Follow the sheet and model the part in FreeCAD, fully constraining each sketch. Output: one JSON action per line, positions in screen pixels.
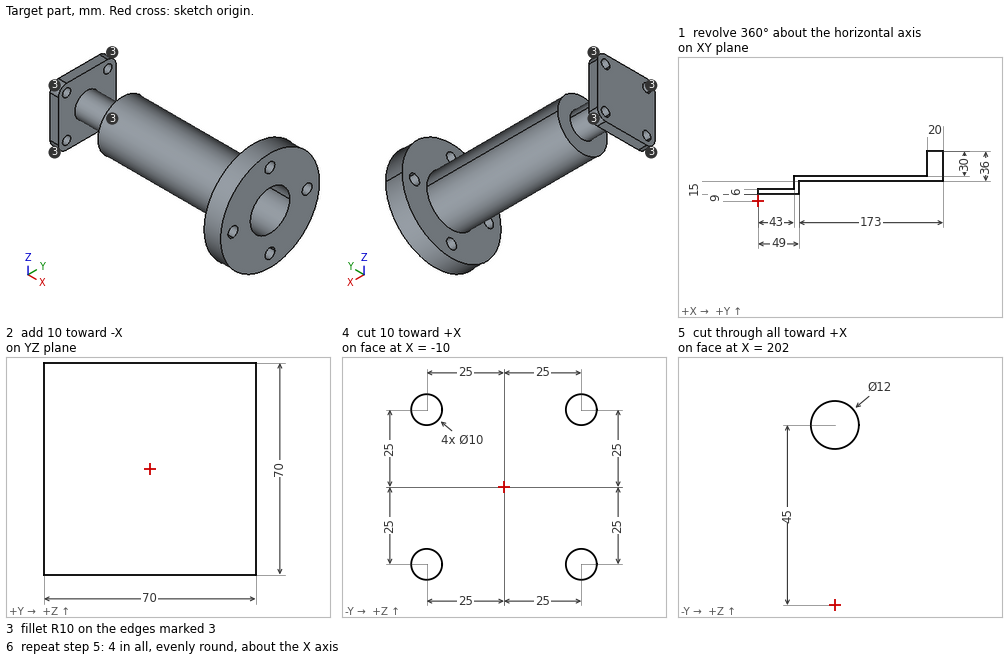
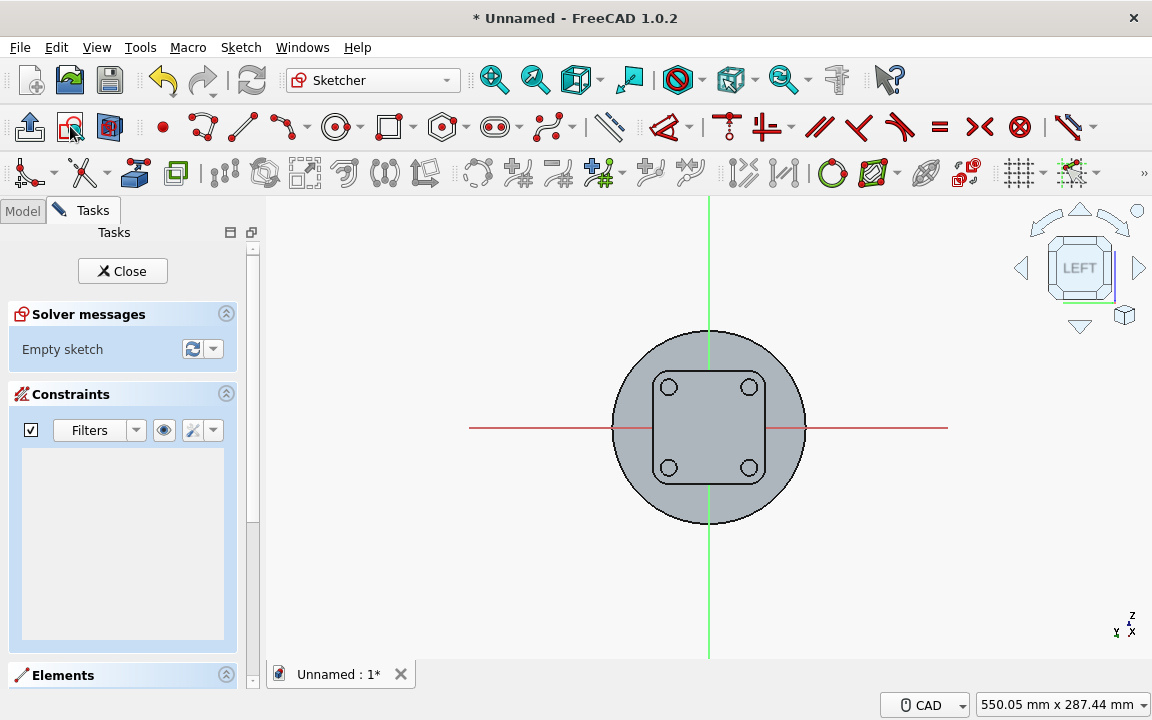
{"action": "scroll", "coordinate": [714, 349], "scroll_direction": "up", "scroll_amount": 13}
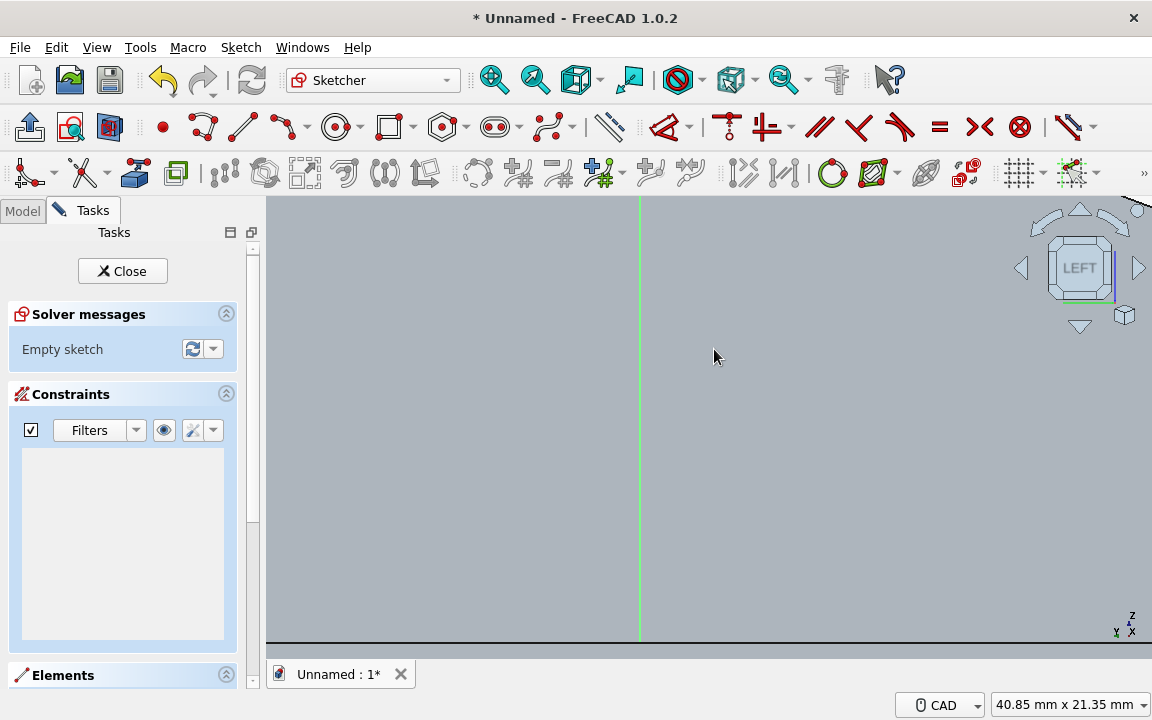
{"action": "key", "text": "g c"}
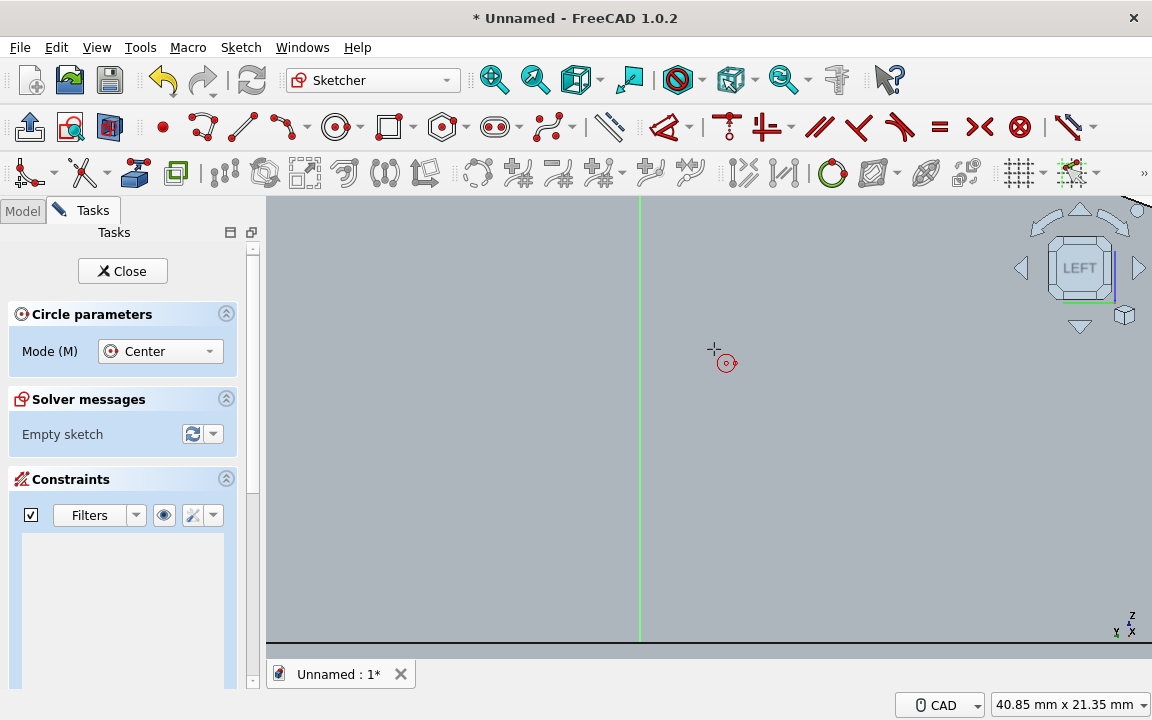
{"action": "left_click", "coordinate": [640, 426]}
{"action": "mouse_move", "coordinate": [732, 334]}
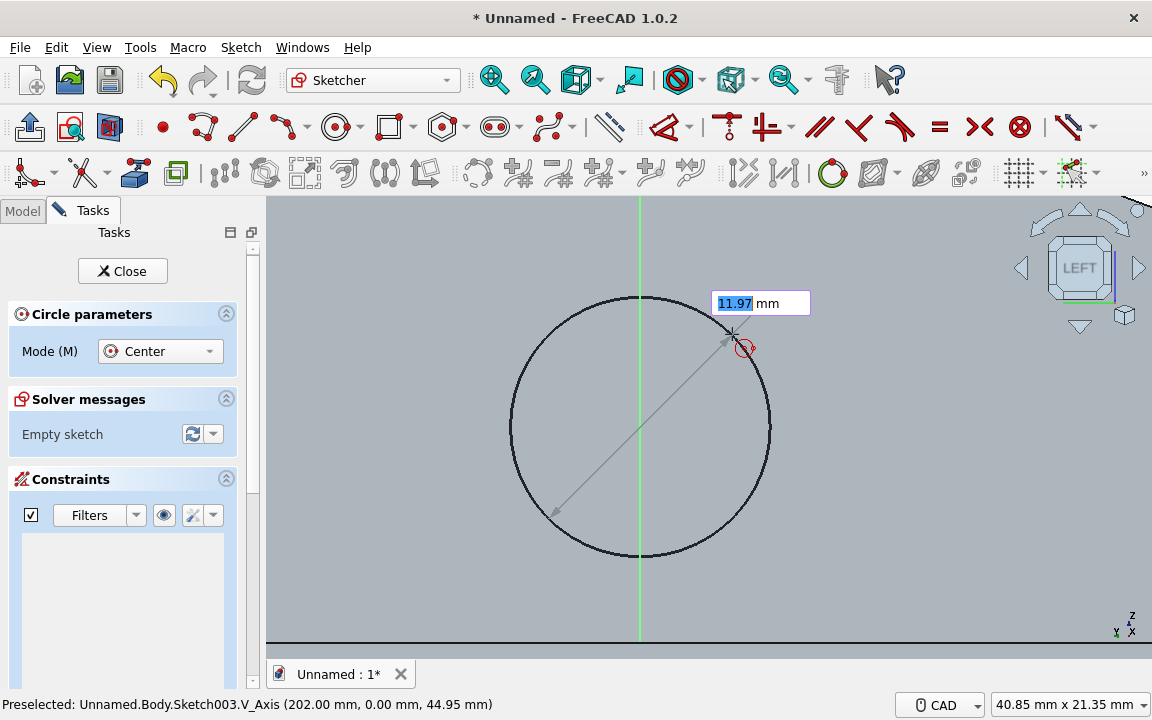
{"action": "type", "text": "12"}
{"action": "key", "text": "Return"}
{"action": "key", "text": "Escape"}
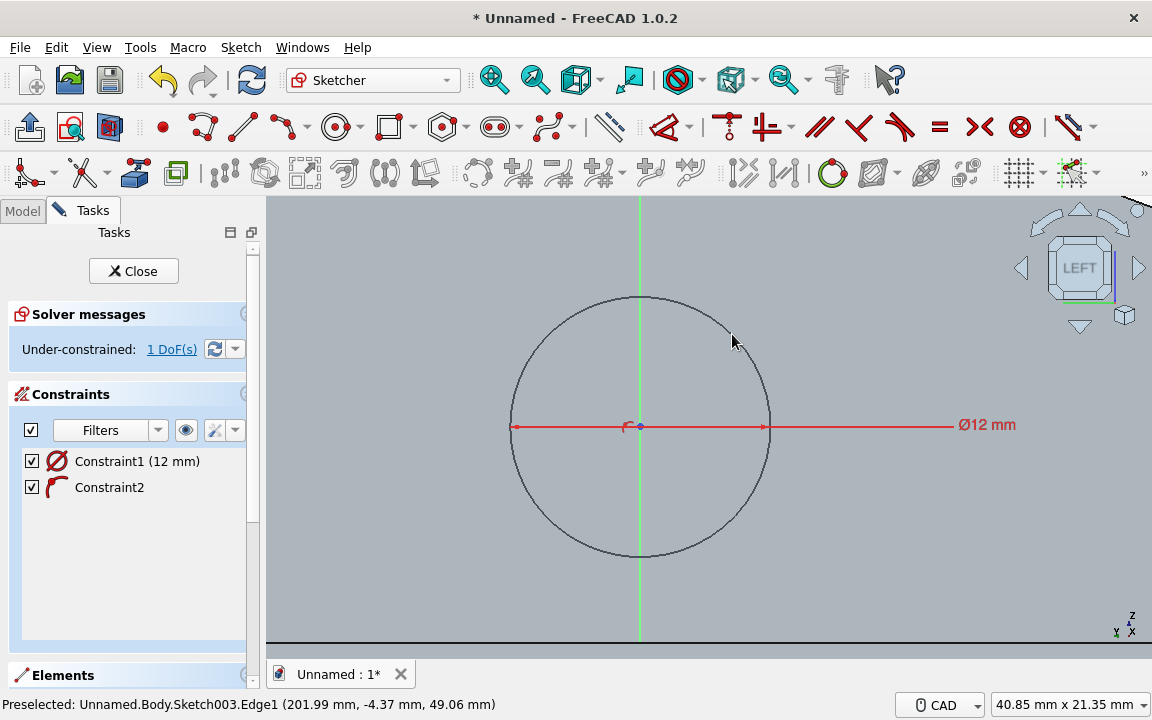
{"action": "left_click", "coordinate": [664, 128]}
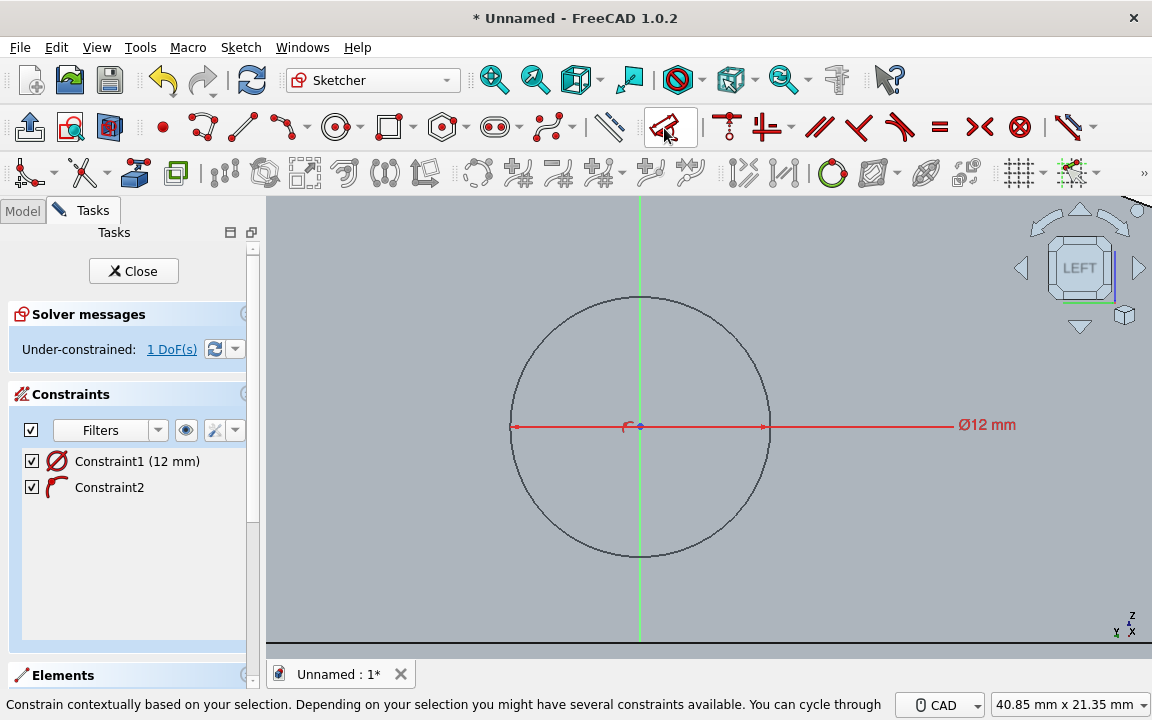
{"action": "left_click", "coordinate": [640, 427]}
{"action": "left_click", "coordinate": [674, 529]}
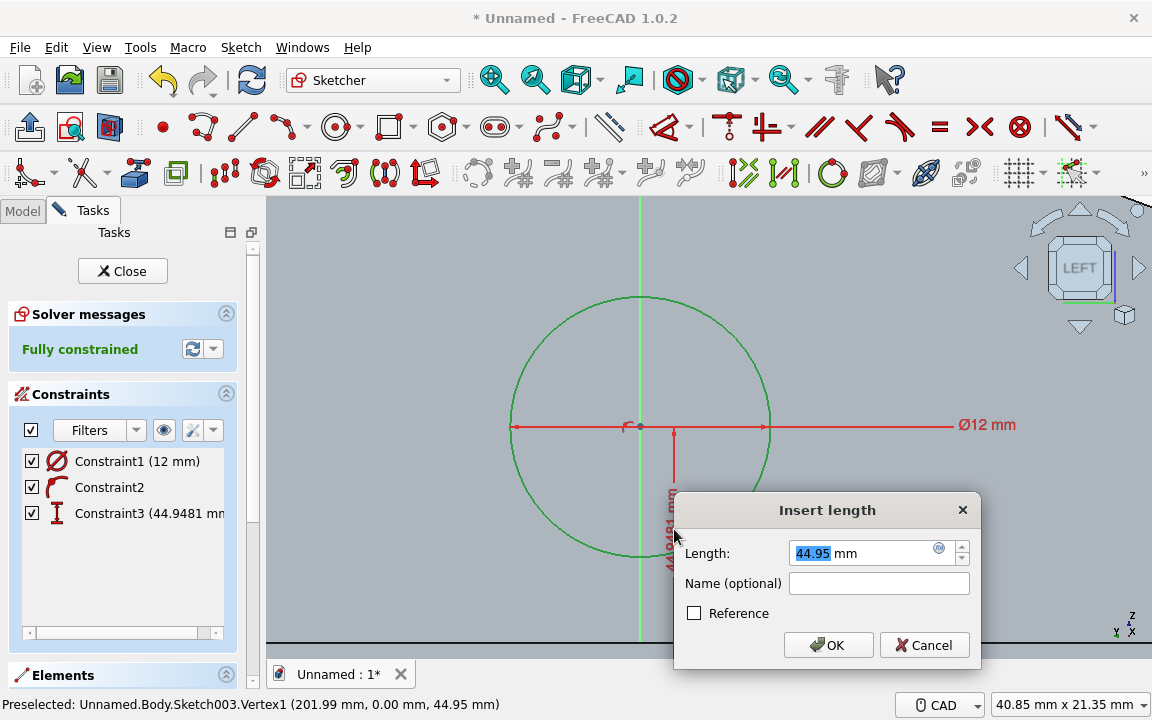
{"action": "type", "text": "45"}
{"action": "key", "text": "Return"}
{"action": "key", "text": "Escape"}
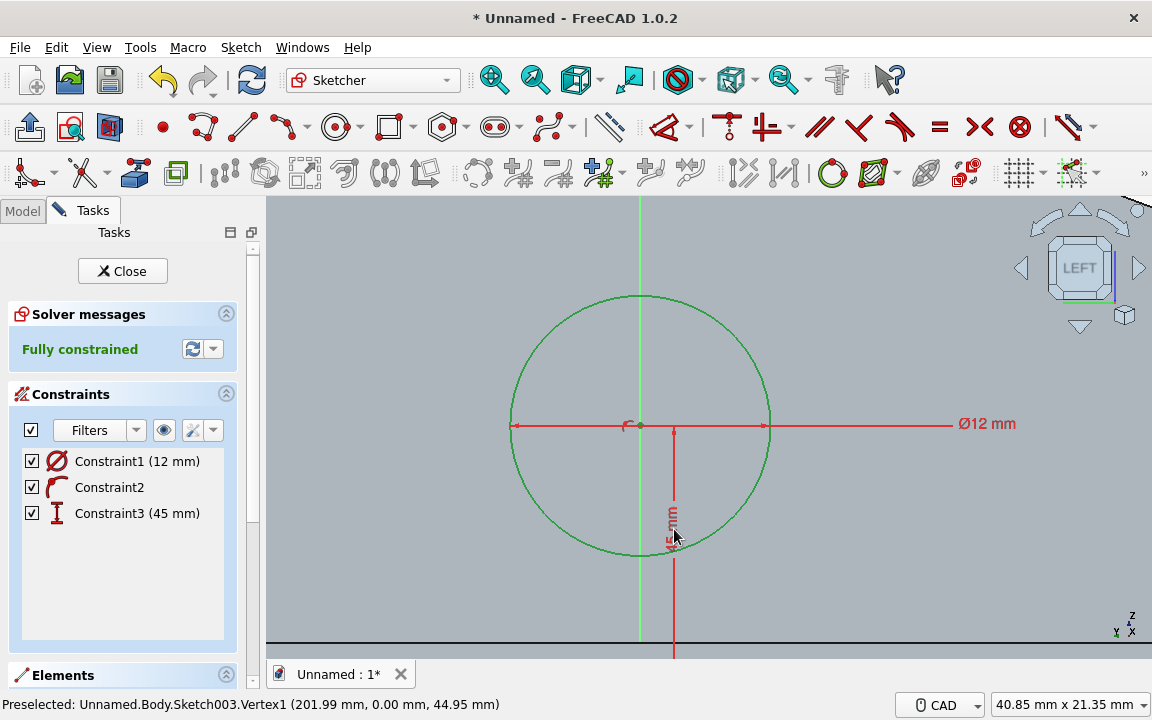
{"action": "left_click", "coordinate": [123, 271]}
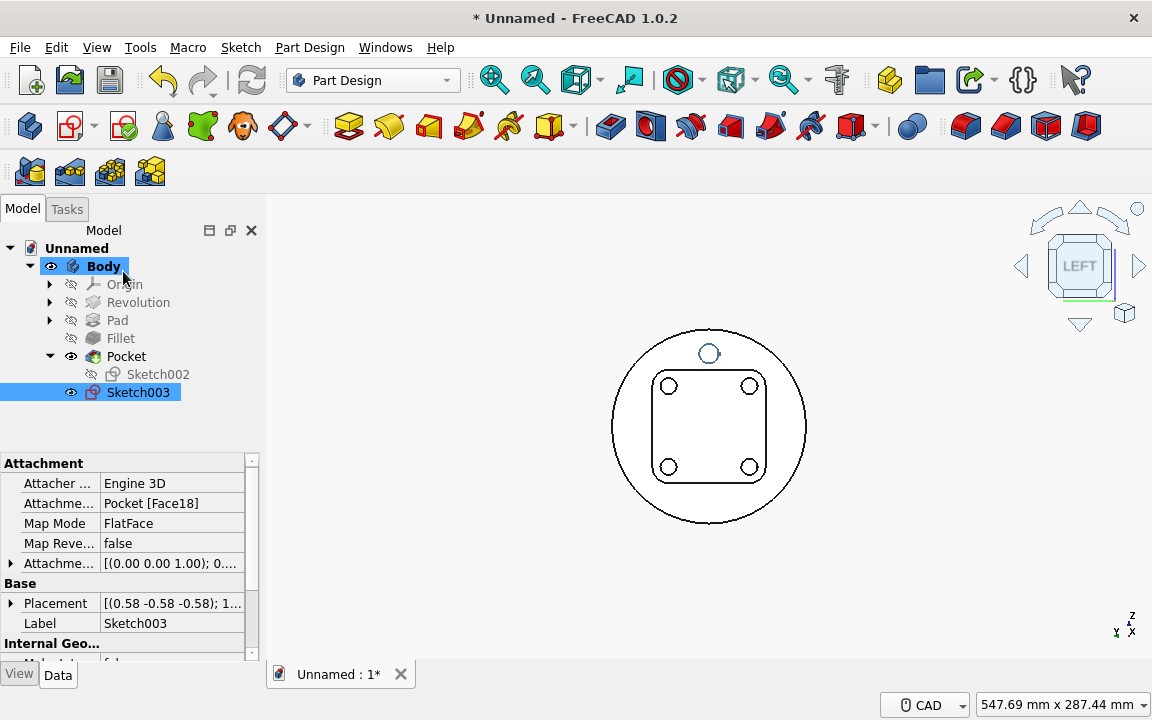
{"action": "left_click", "coordinate": [612, 126]}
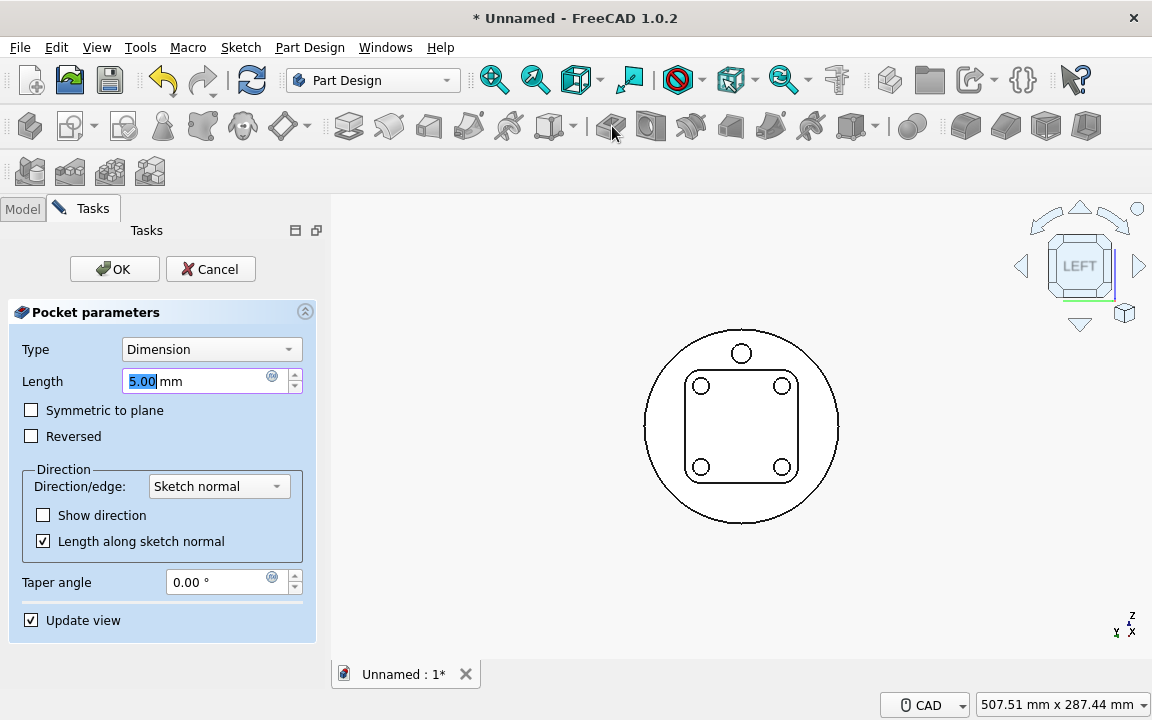
{"action": "left_click", "coordinate": [212, 350]}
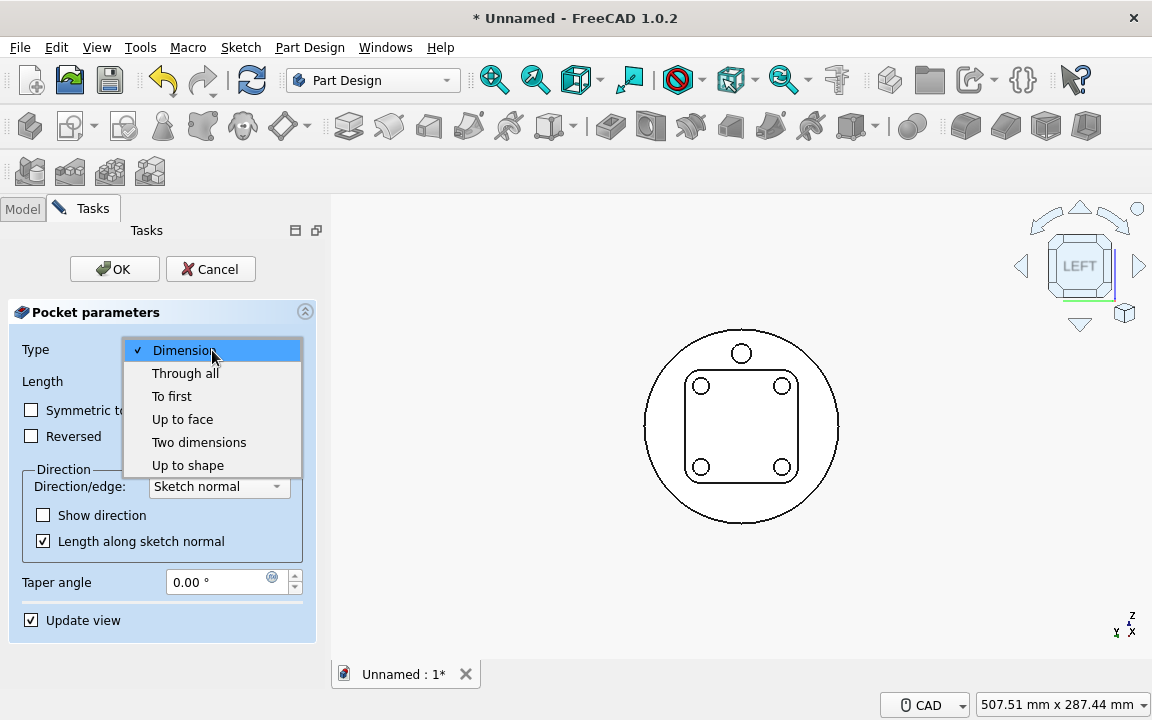
{"action": "left_click", "coordinate": [212, 374]}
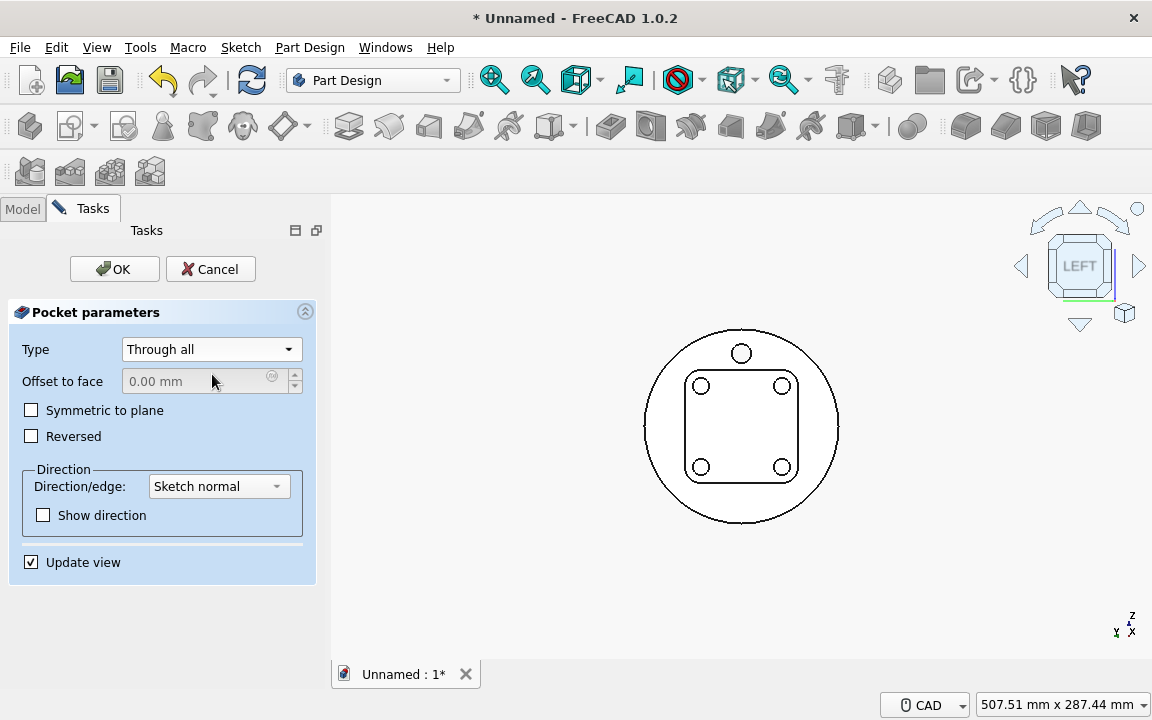
{"action": "left_click", "coordinate": [115, 269]}